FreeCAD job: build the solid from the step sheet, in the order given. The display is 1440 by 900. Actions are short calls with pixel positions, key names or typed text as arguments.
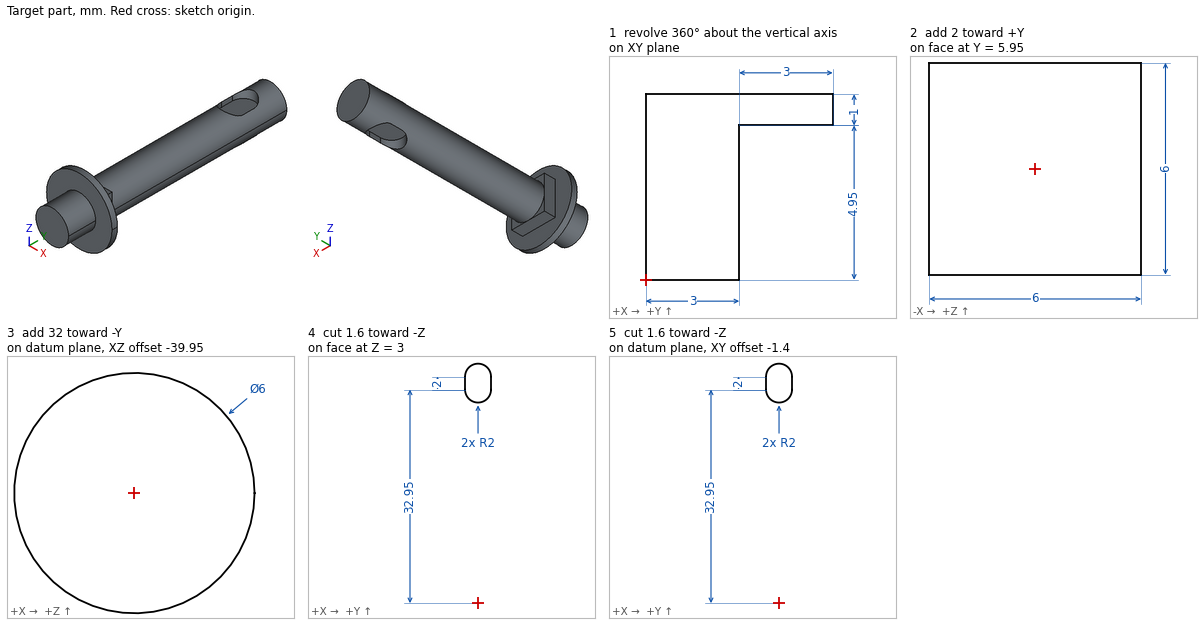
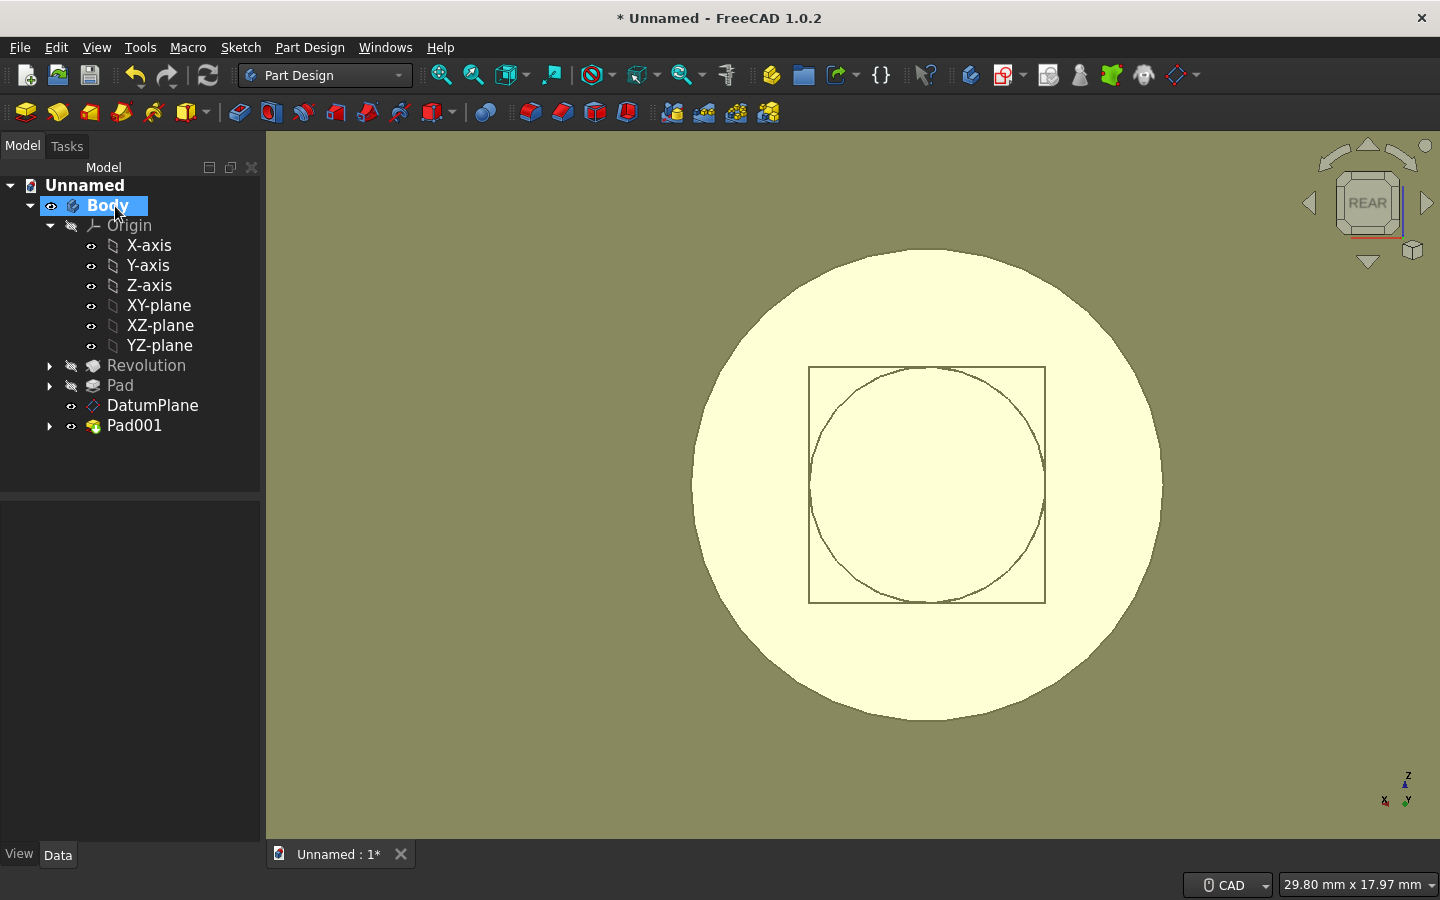
click(116, 406)
key(space)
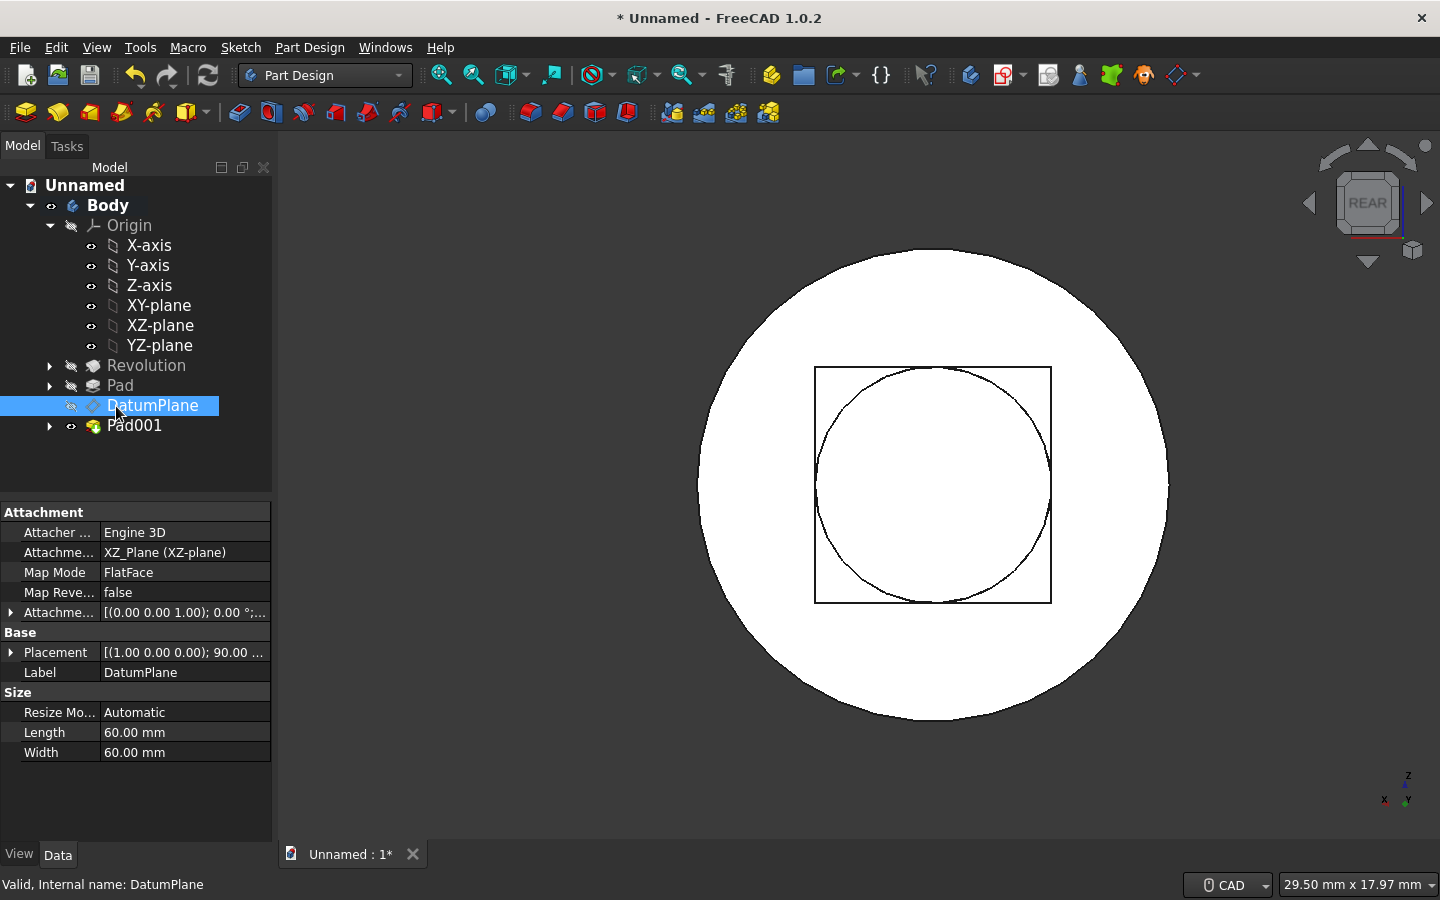
key(0)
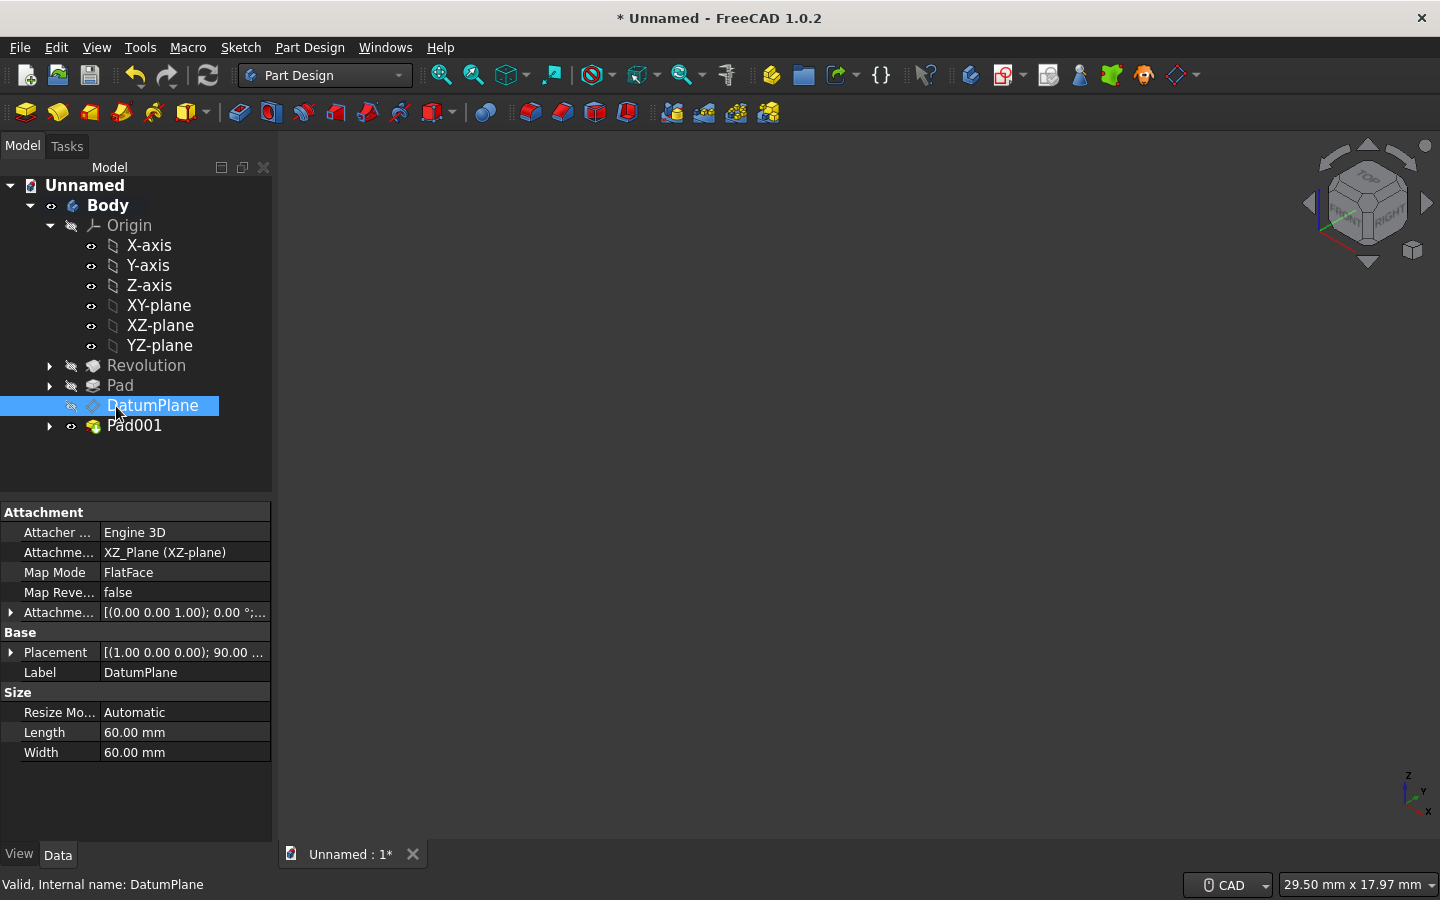
click(442, 76)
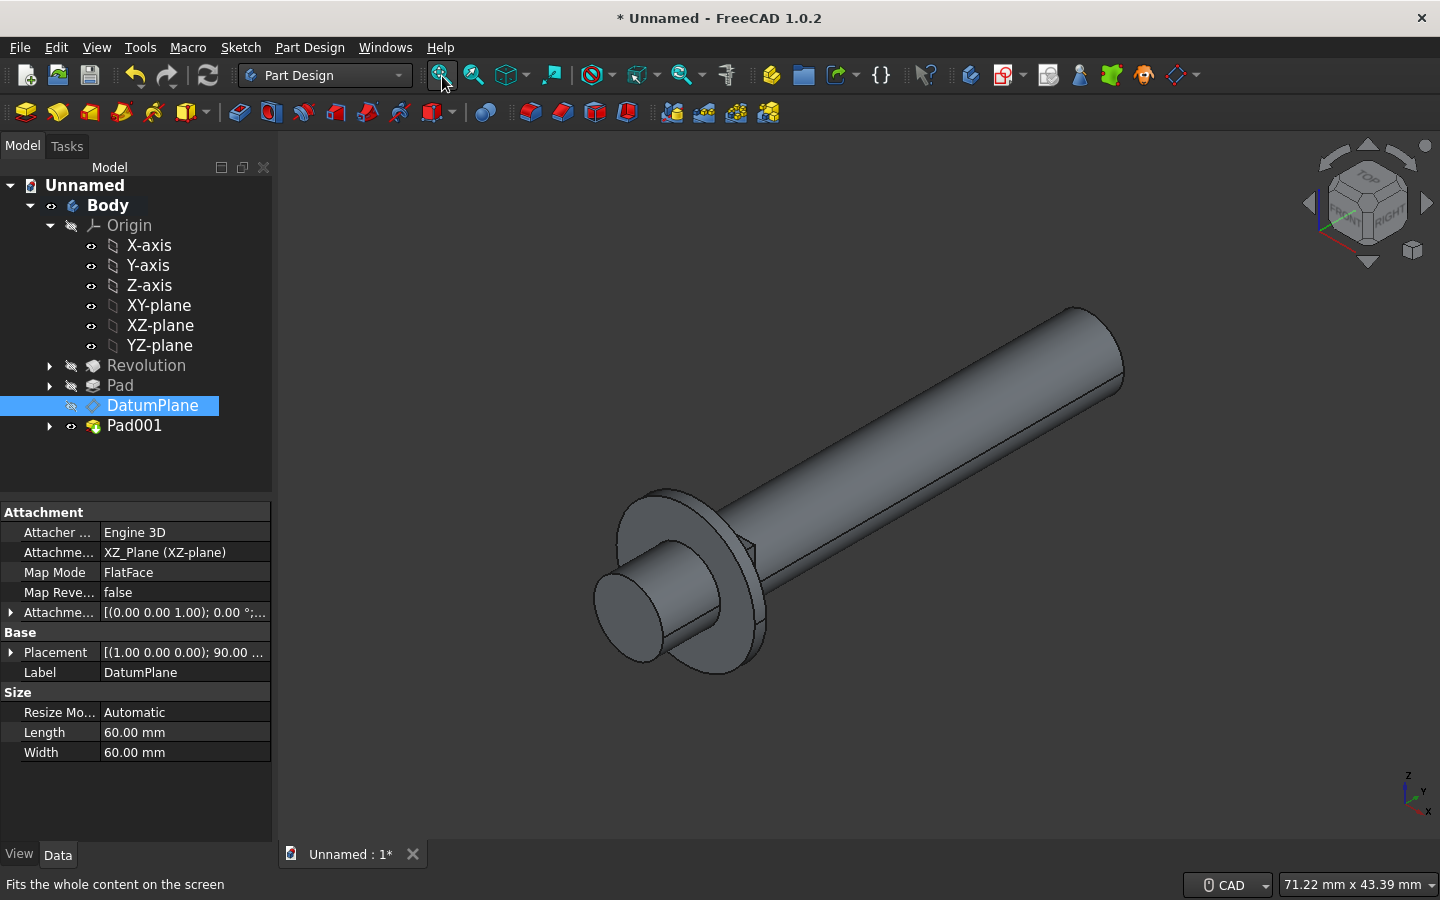
key(2)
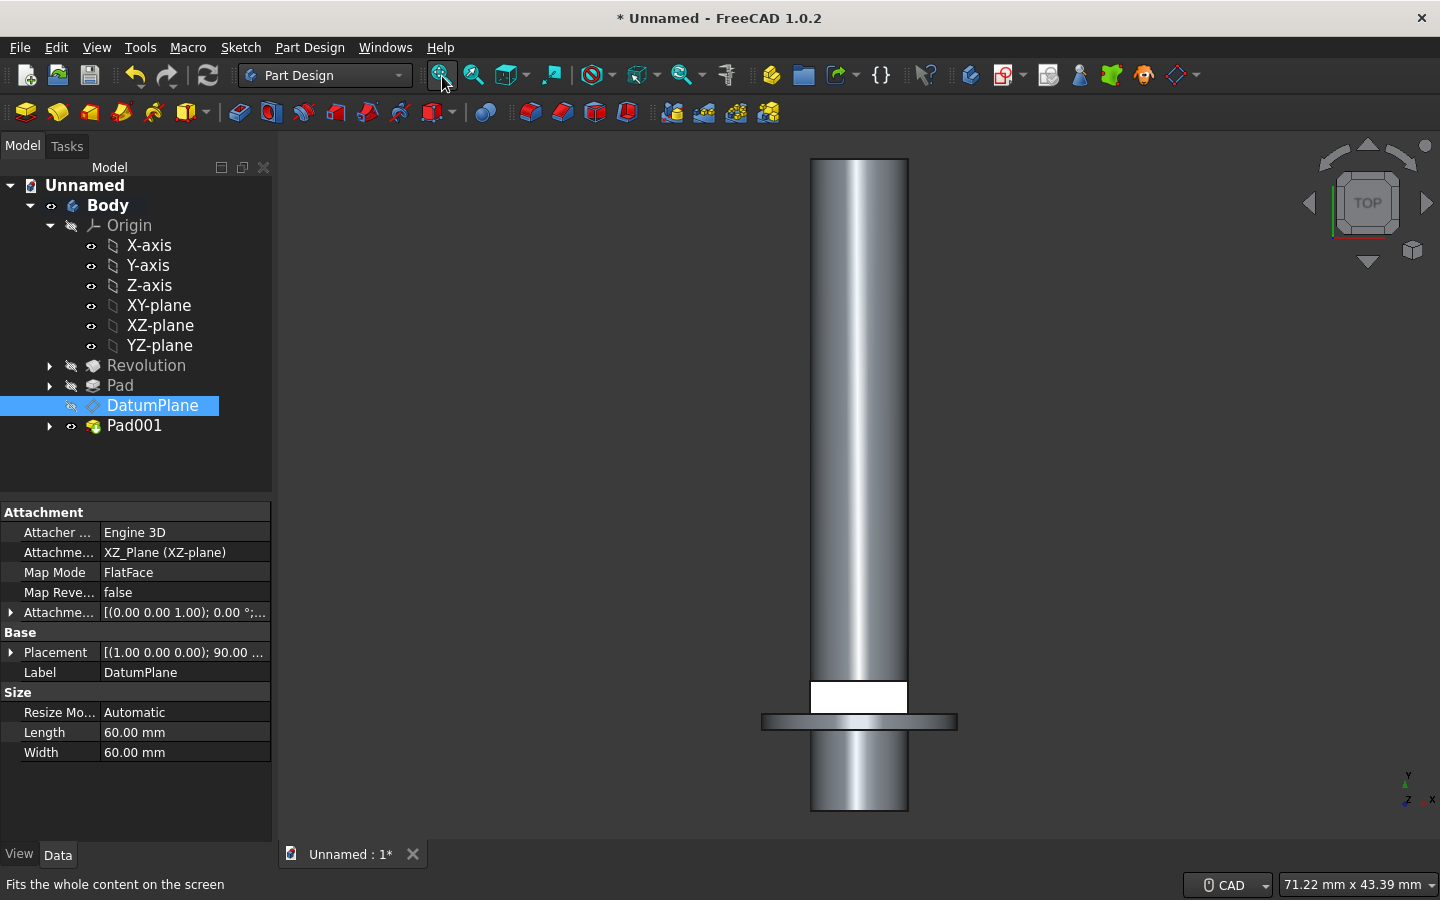
click(887, 697)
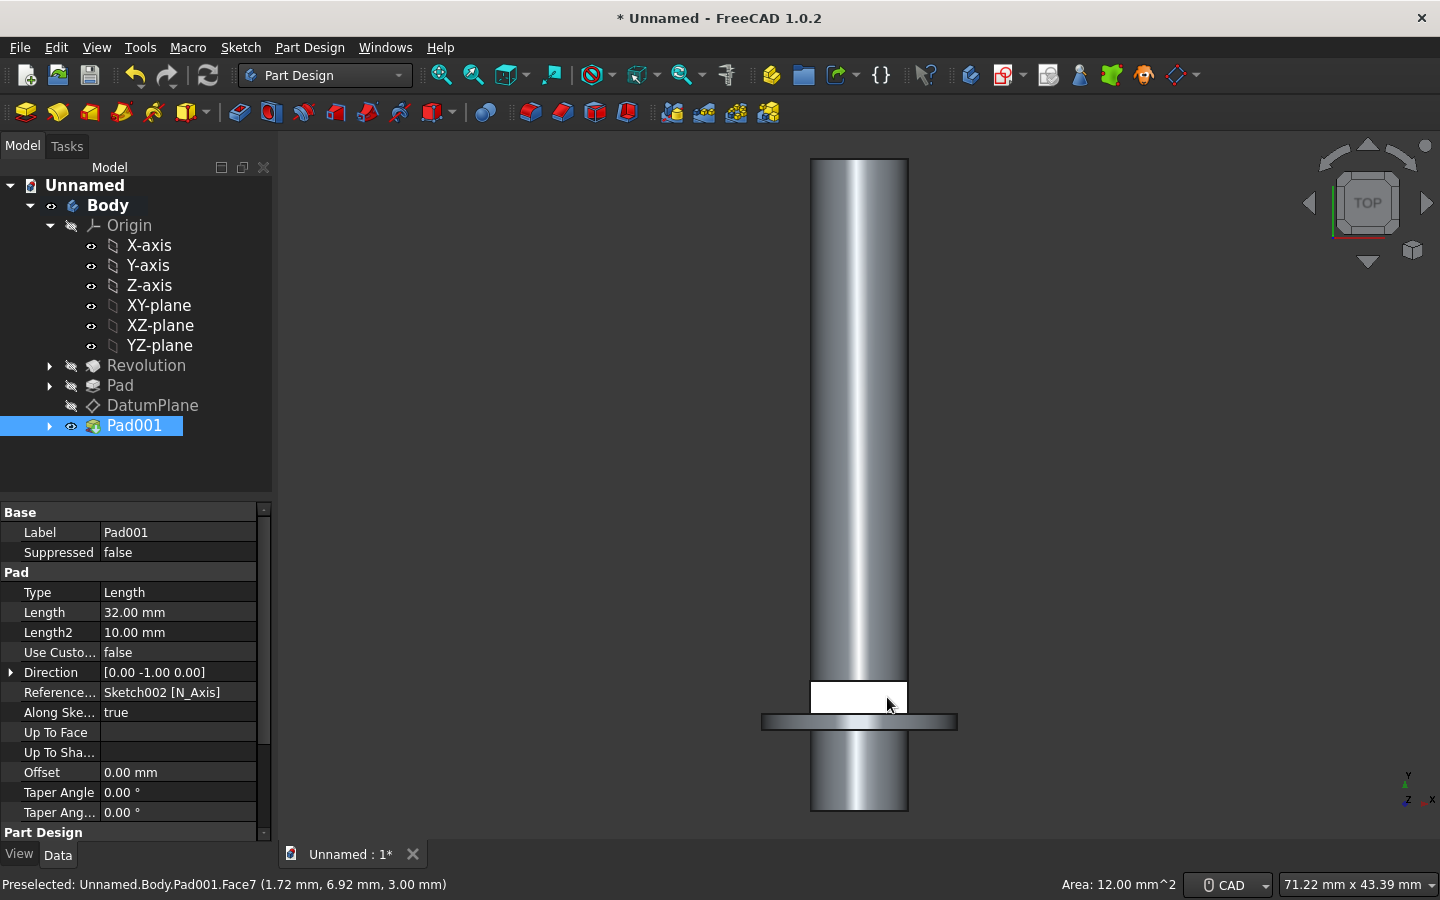
click(1004, 76)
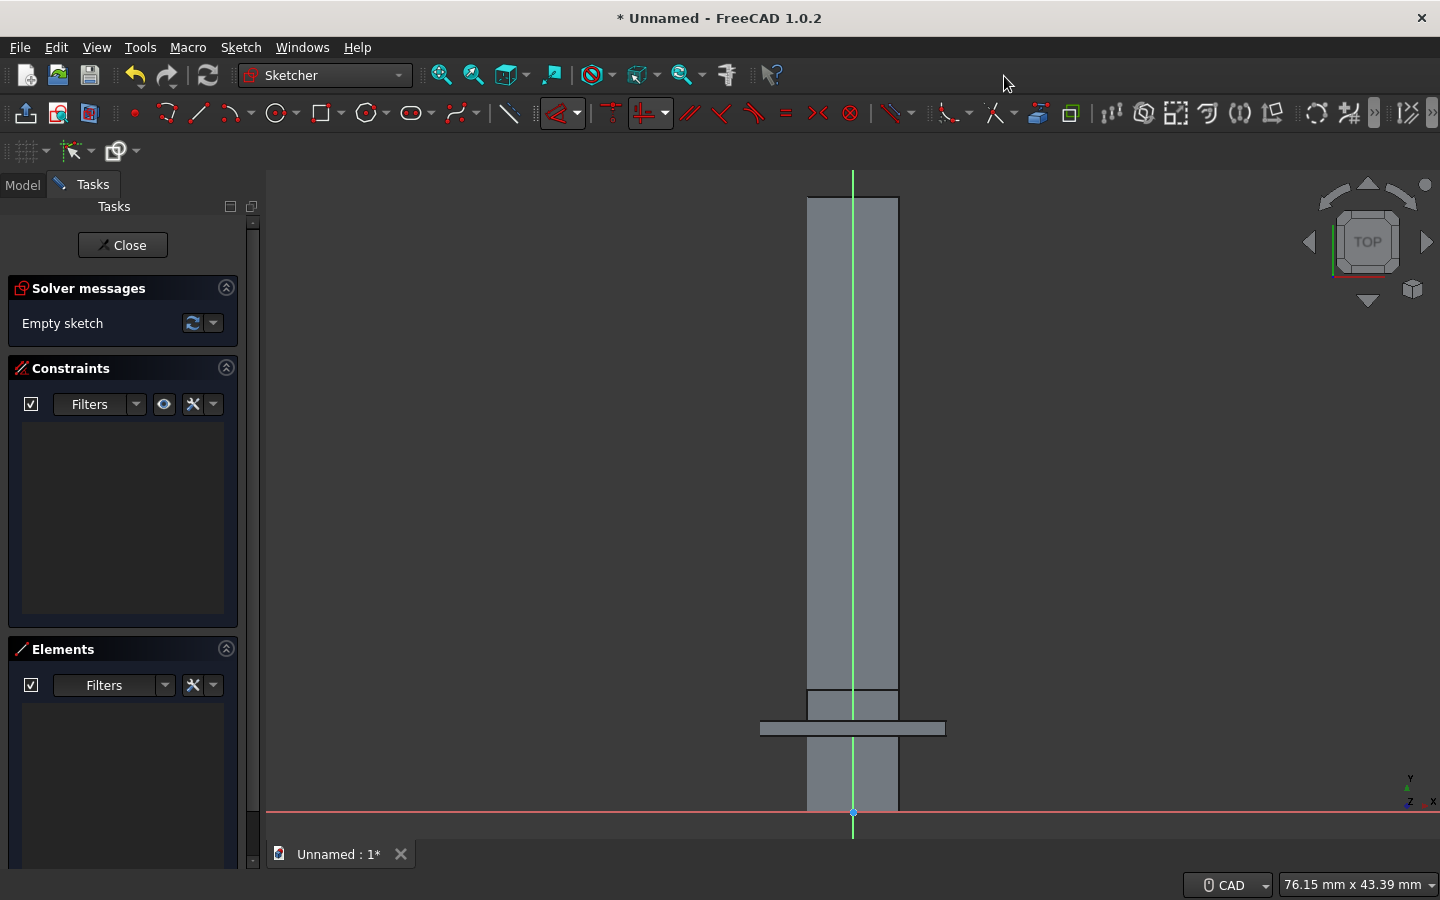
scroll(870, 235, up, 8)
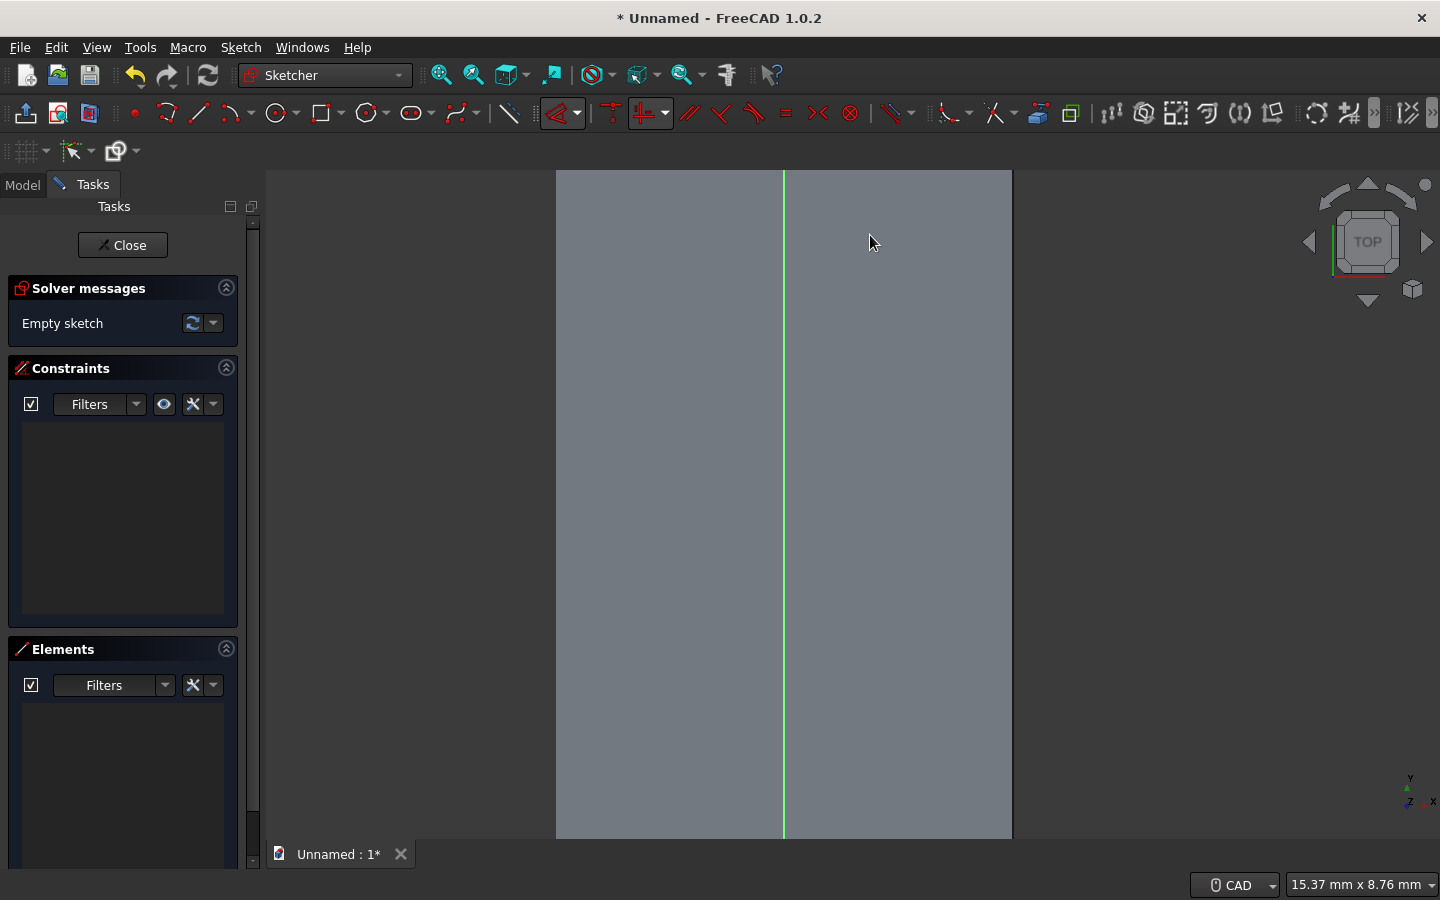
click(412, 114)